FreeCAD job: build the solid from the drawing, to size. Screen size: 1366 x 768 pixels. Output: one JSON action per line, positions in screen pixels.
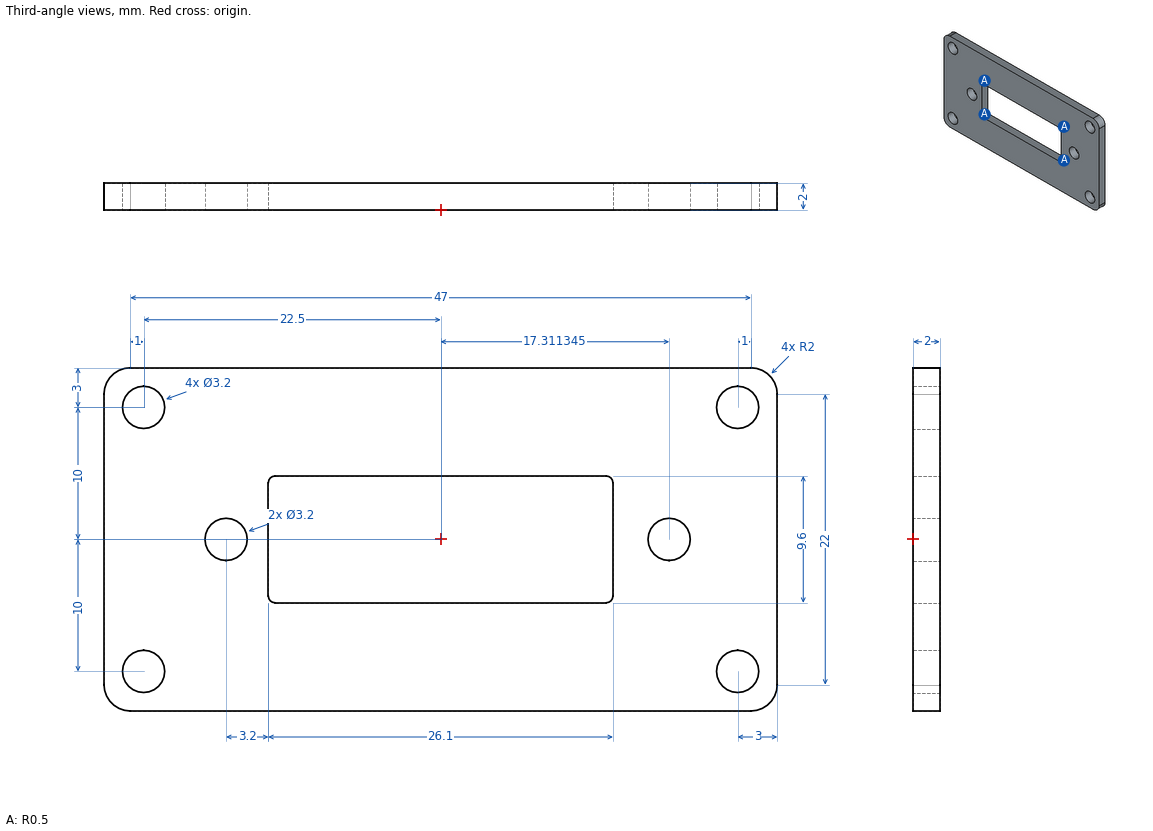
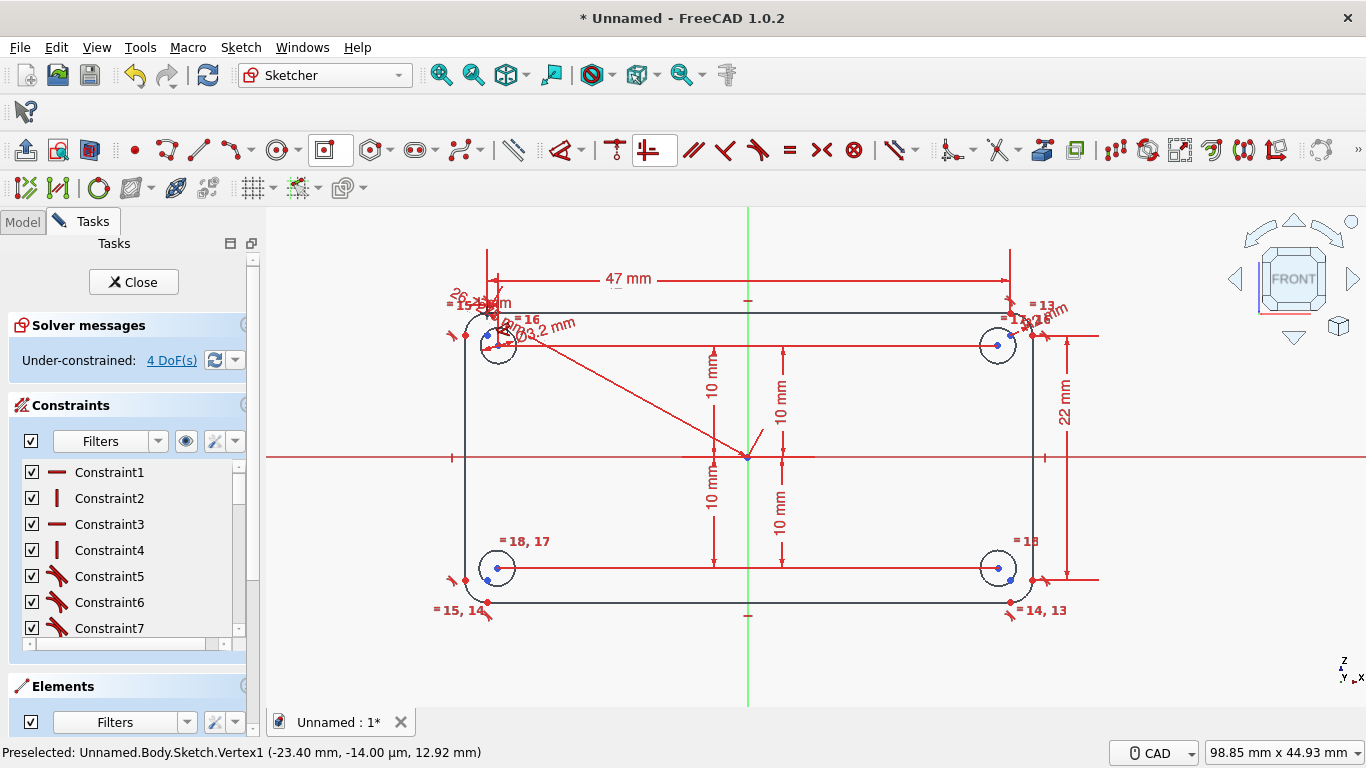
{"action": "left_click", "coordinate": [498, 346]}
{"action": "left_click", "coordinate": [429, 330]}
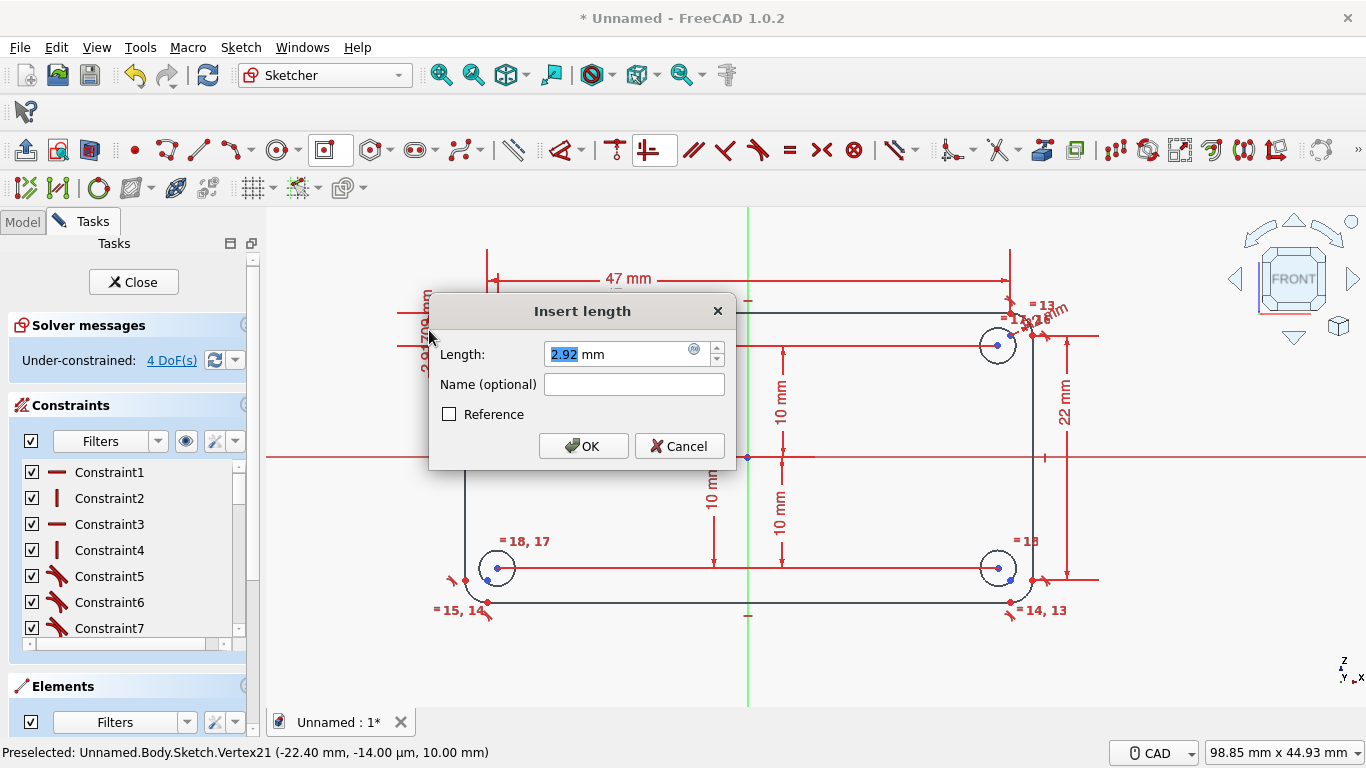
{"action": "type", "text": "3"}
{"action": "key", "text": "Return"}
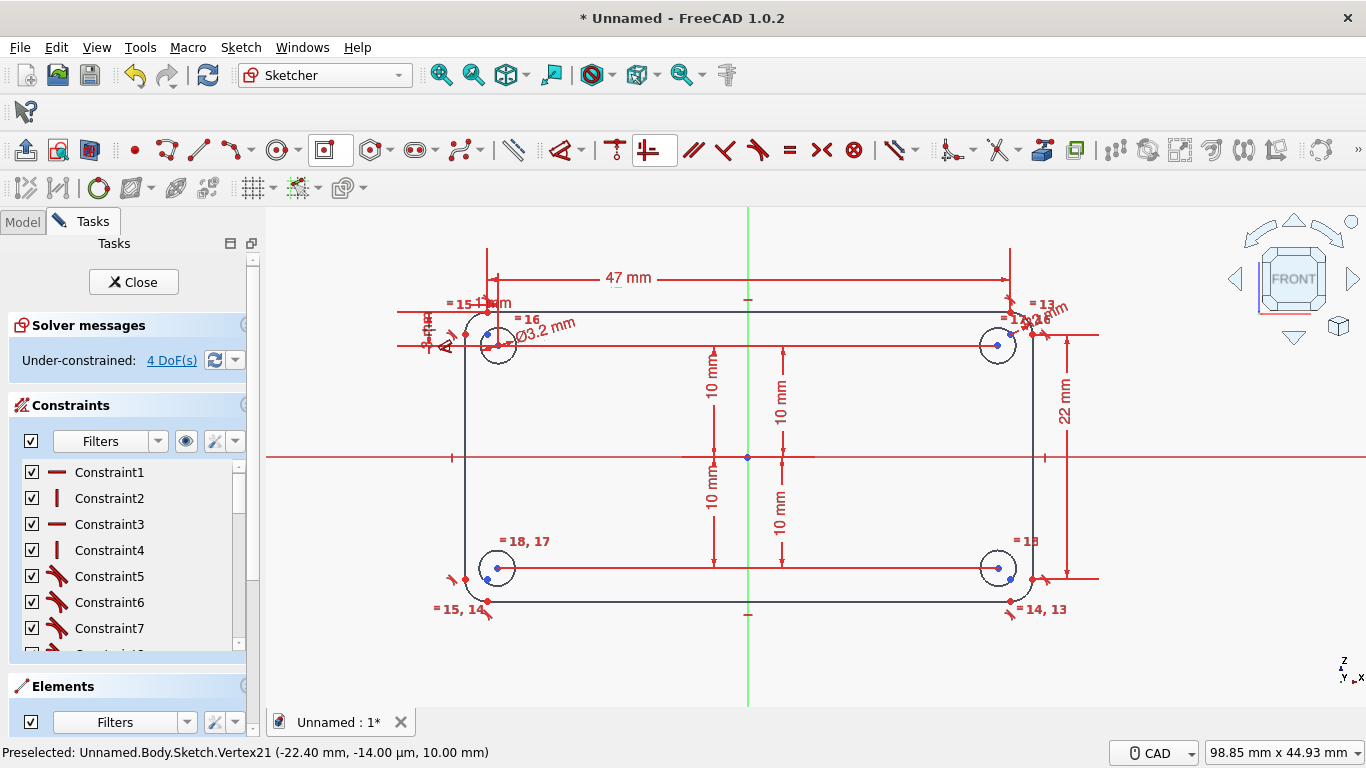
{"action": "scroll", "coordinate": [1010, 312], "scroll_direction": "up", "scroll_amount": 7}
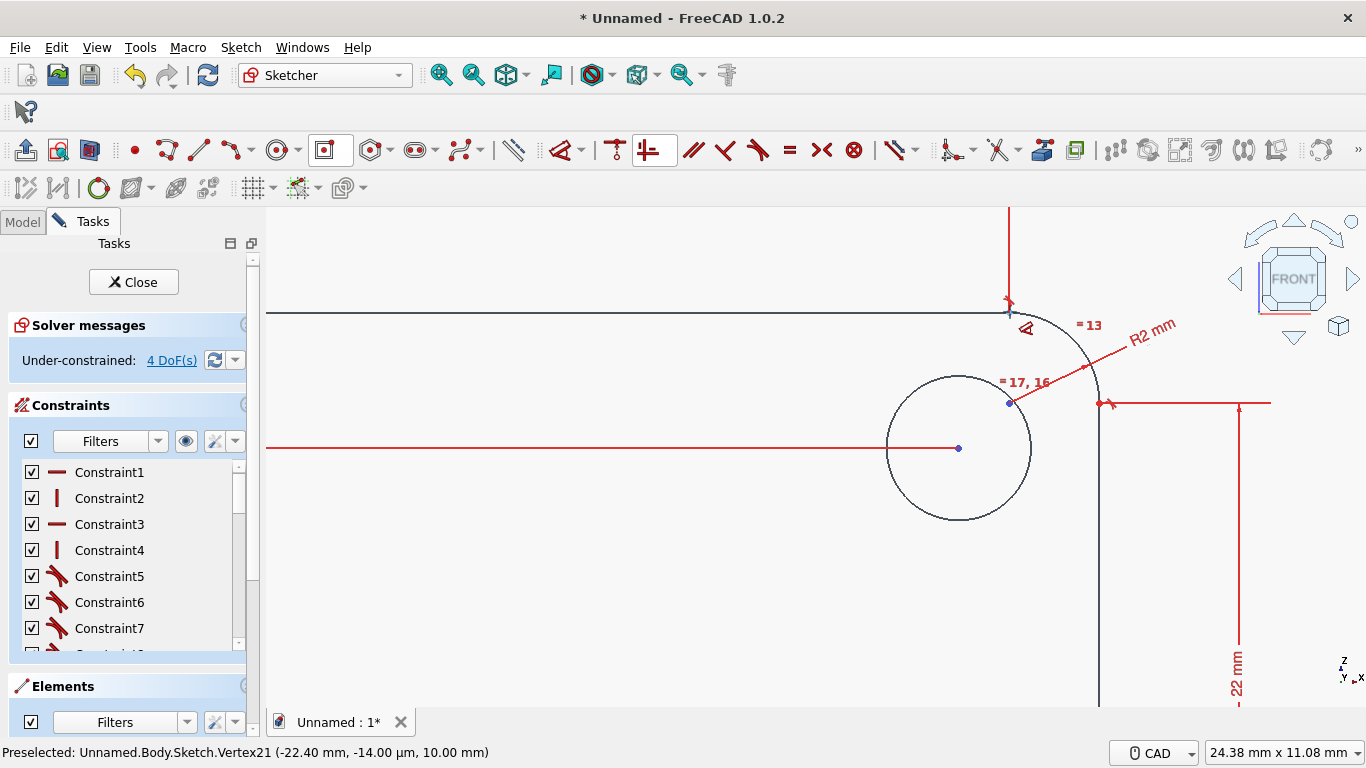
{"action": "left_click", "coordinate": [1009, 313]}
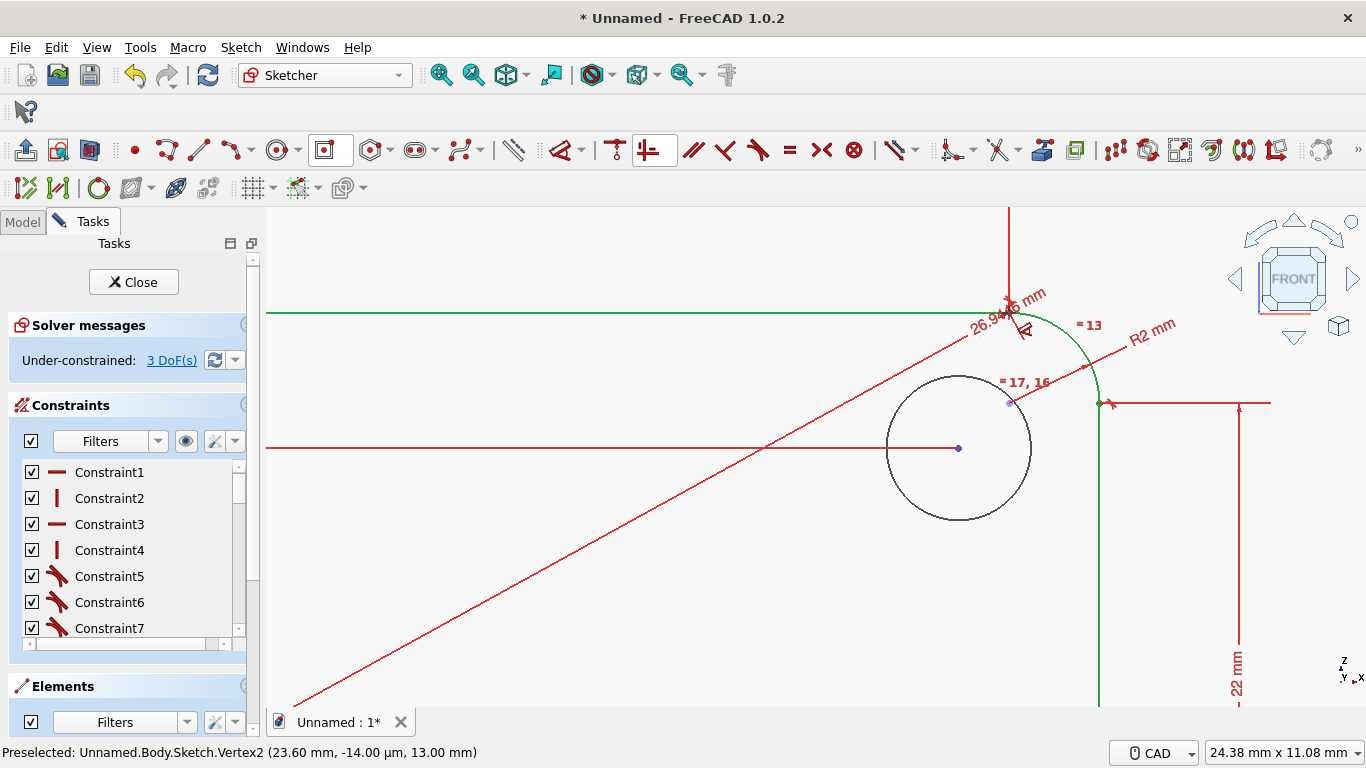
{"action": "left_click", "coordinate": [959, 448]}
{"action": "left_click", "coordinate": [984, 279]}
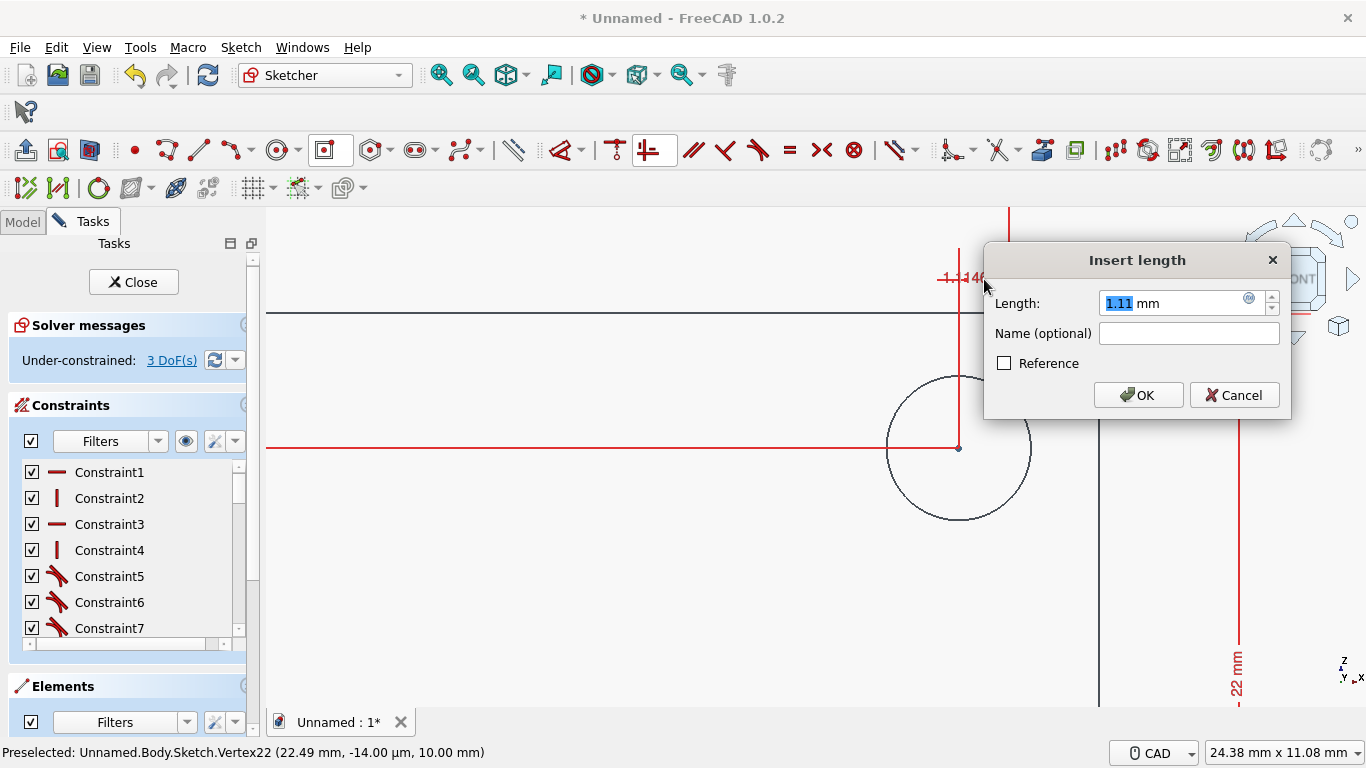
{"action": "type", "text": "1"}
{"action": "key", "text": "Return"}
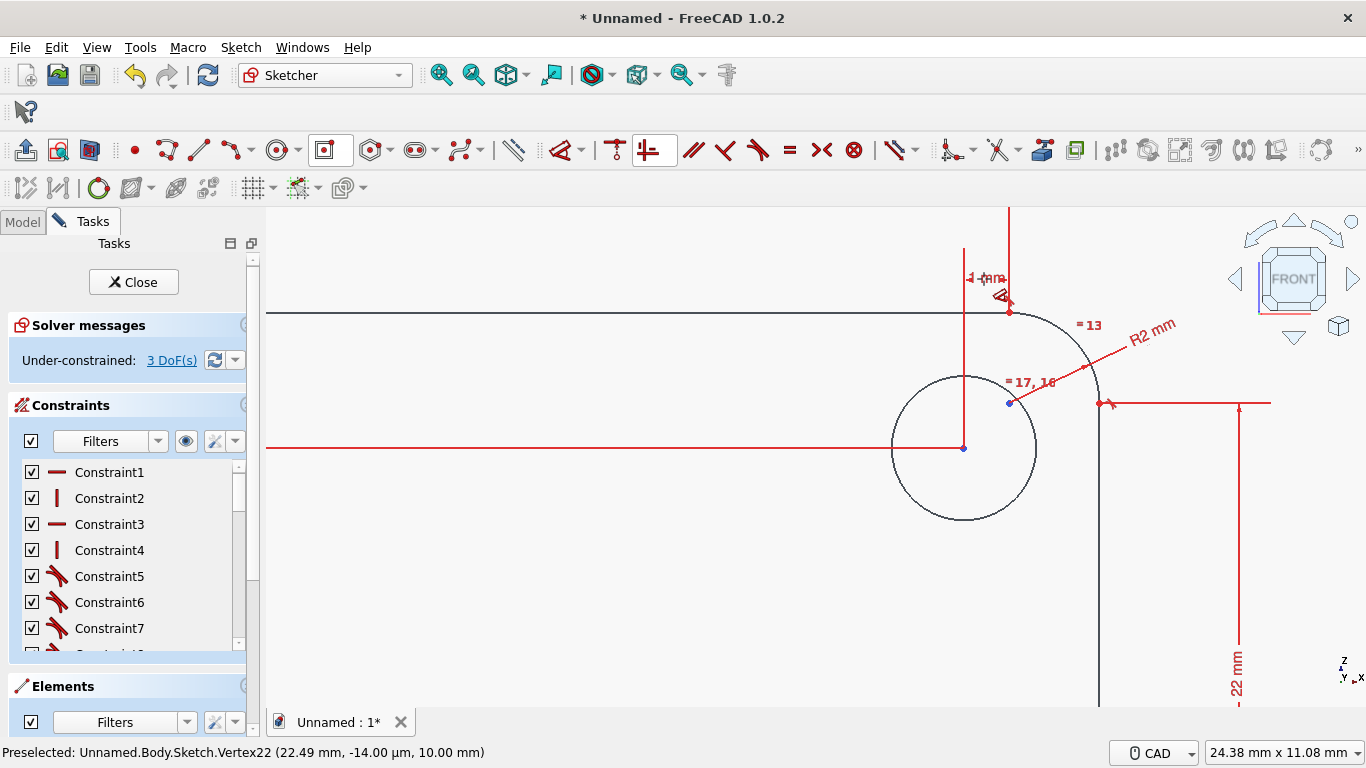
{"action": "scroll", "coordinate": [1010, 312], "scroll_direction": "down", "scroll_amount": 7}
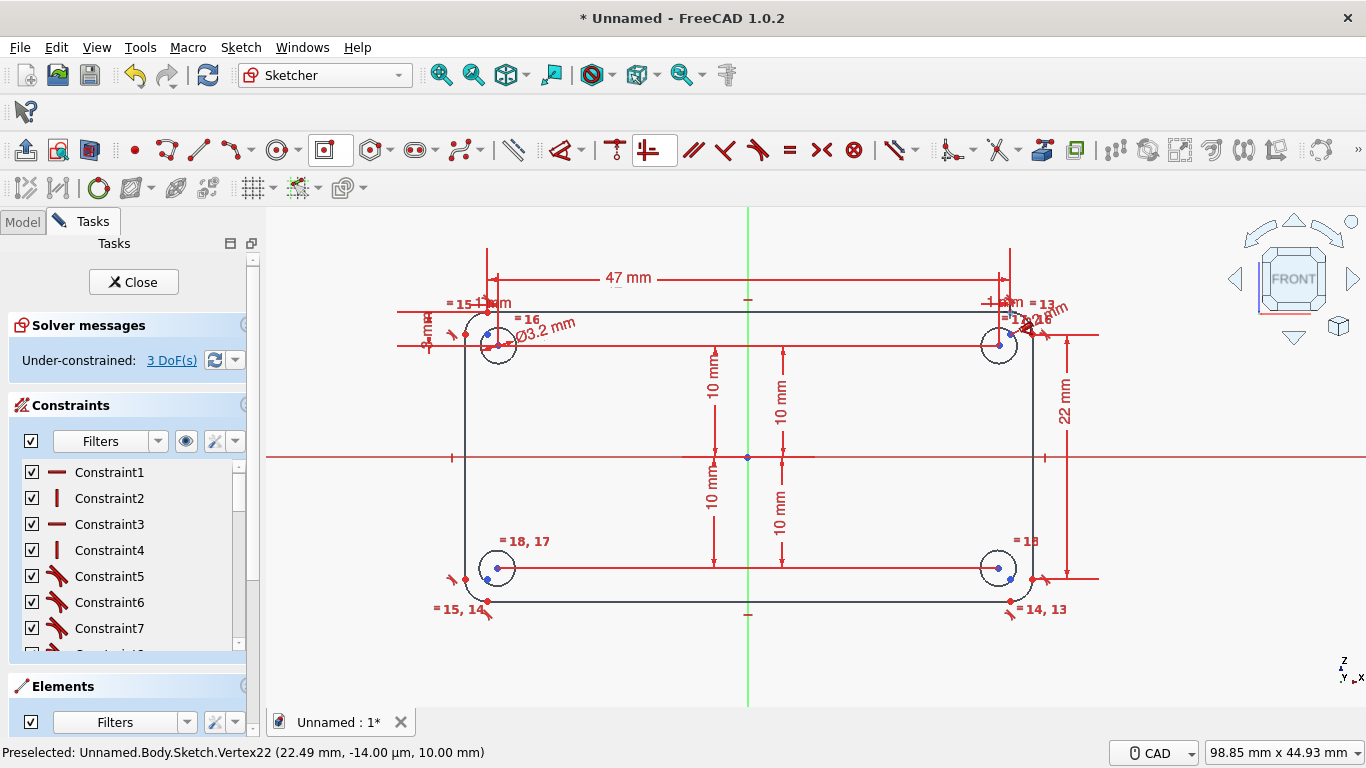
{"action": "scroll", "coordinate": [487, 602], "scroll_direction": "up", "scroll_amount": 7}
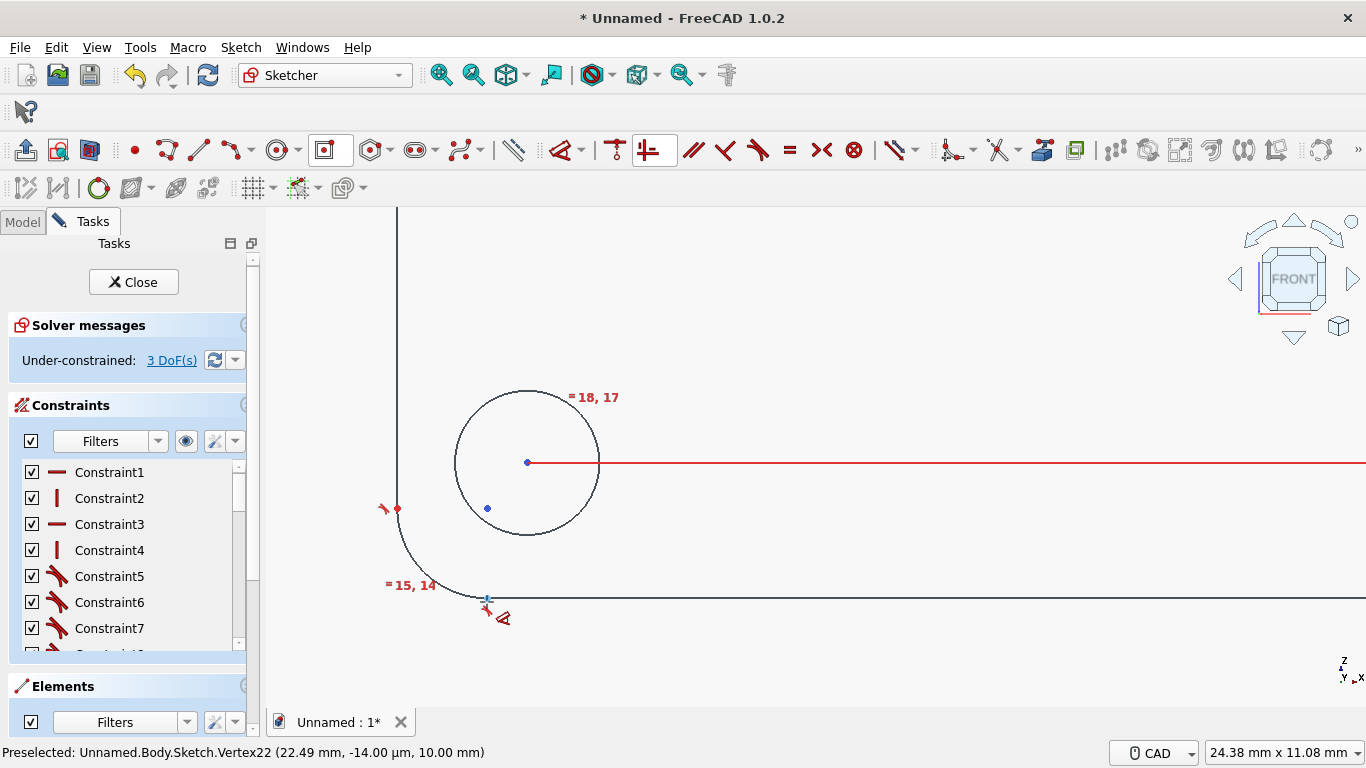
{"action": "left_click", "coordinate": [488, 598]}